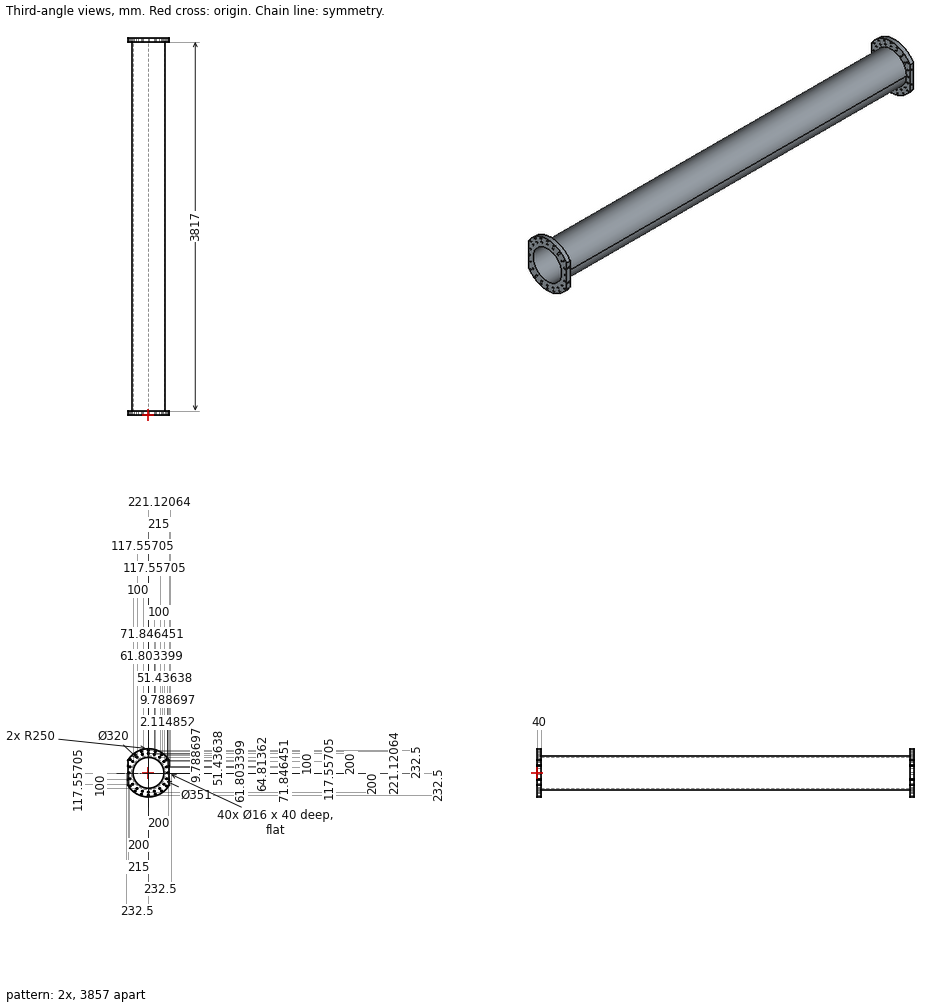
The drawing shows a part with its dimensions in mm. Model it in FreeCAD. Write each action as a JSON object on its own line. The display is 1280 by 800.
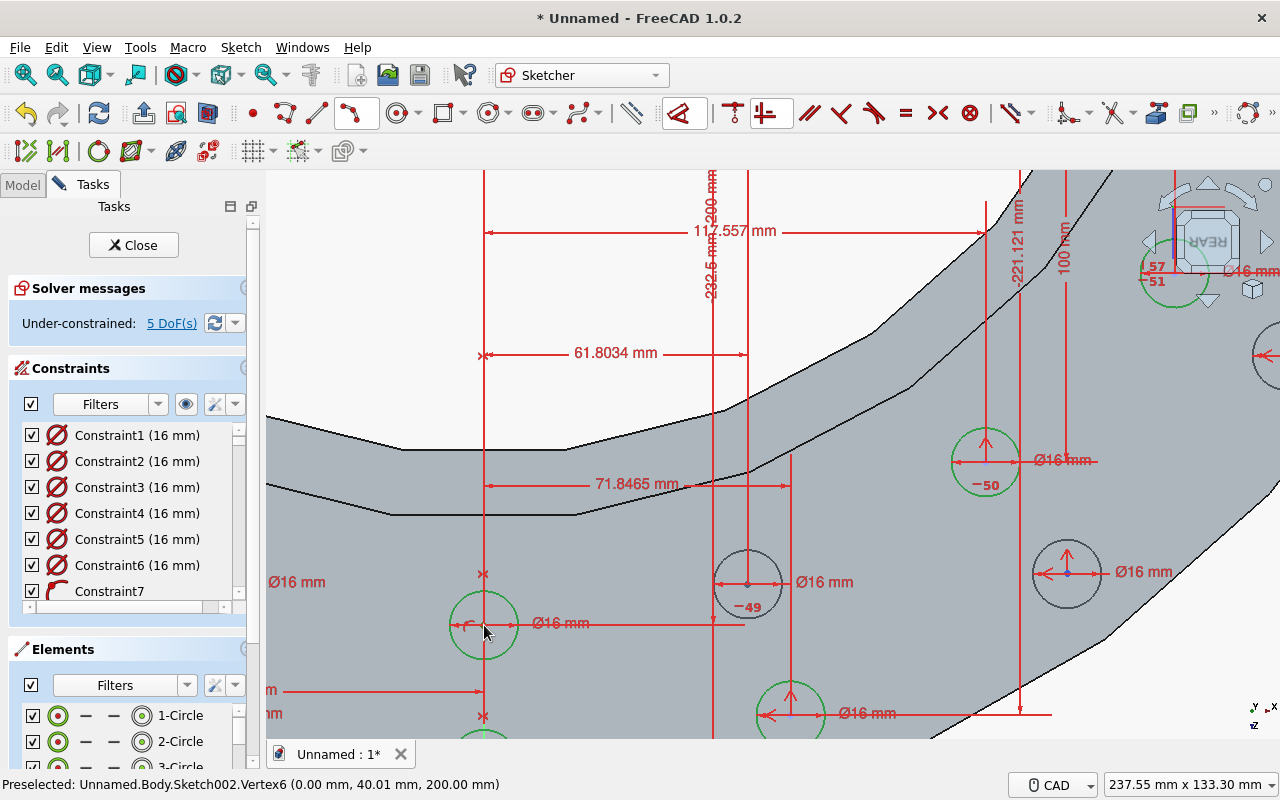
{"action": "key", "text": "i"}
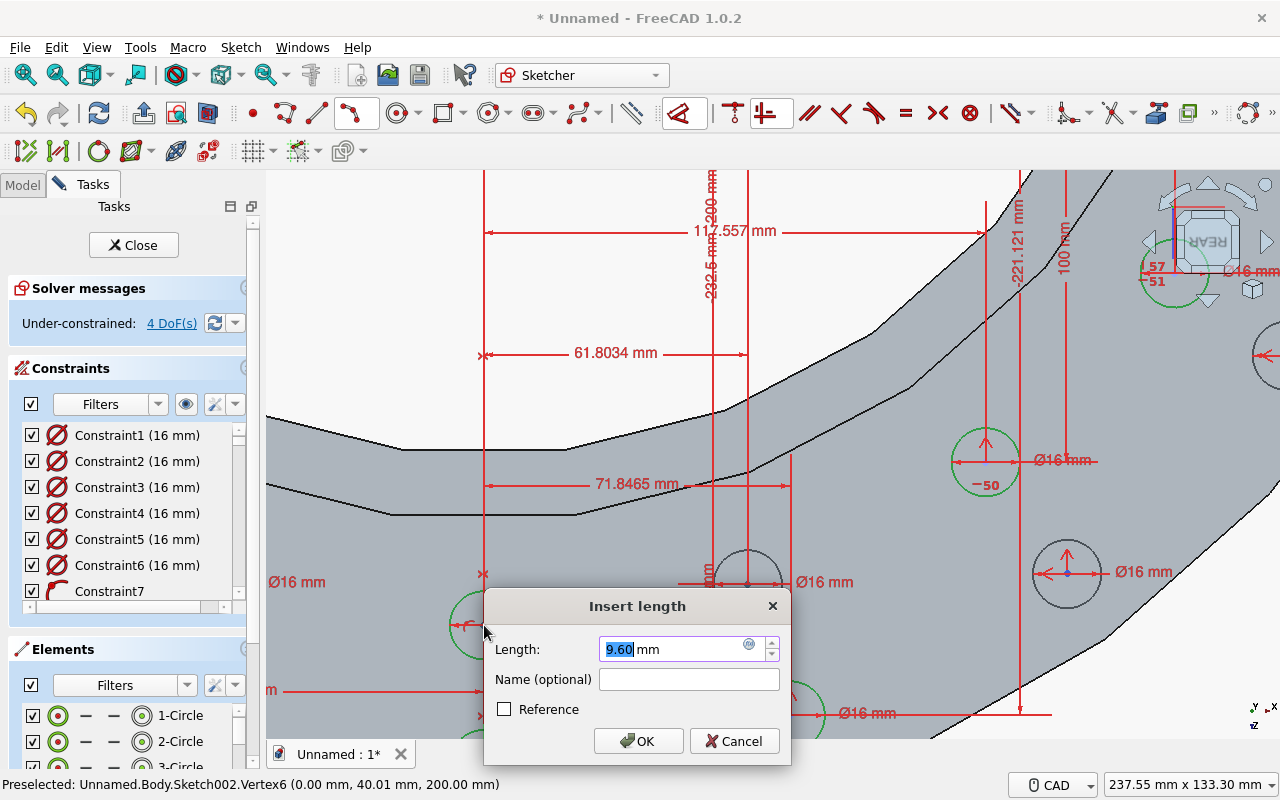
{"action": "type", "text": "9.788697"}
{"action": "key", "text": "Return"}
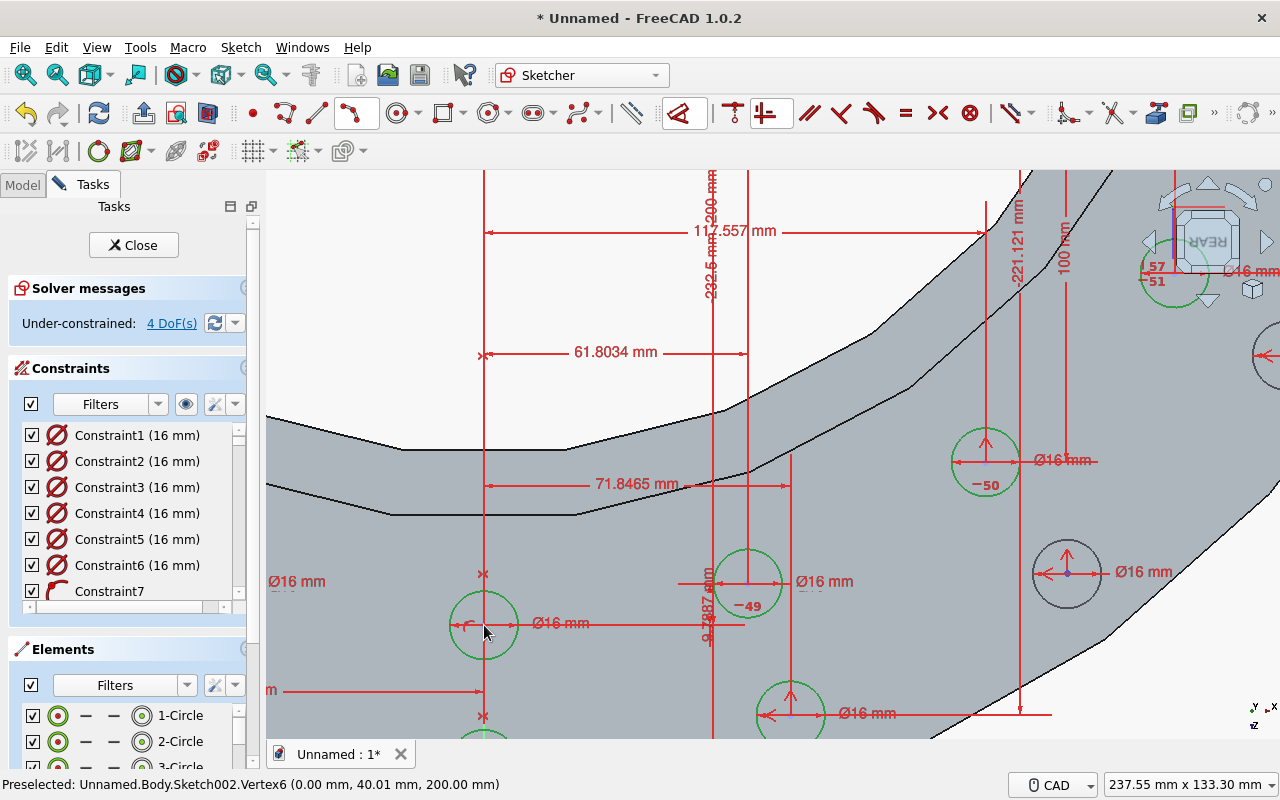
{"action": "scroll", "coordinate": [748, 590], "scroll_direction": "down", "scroll_amount": 9}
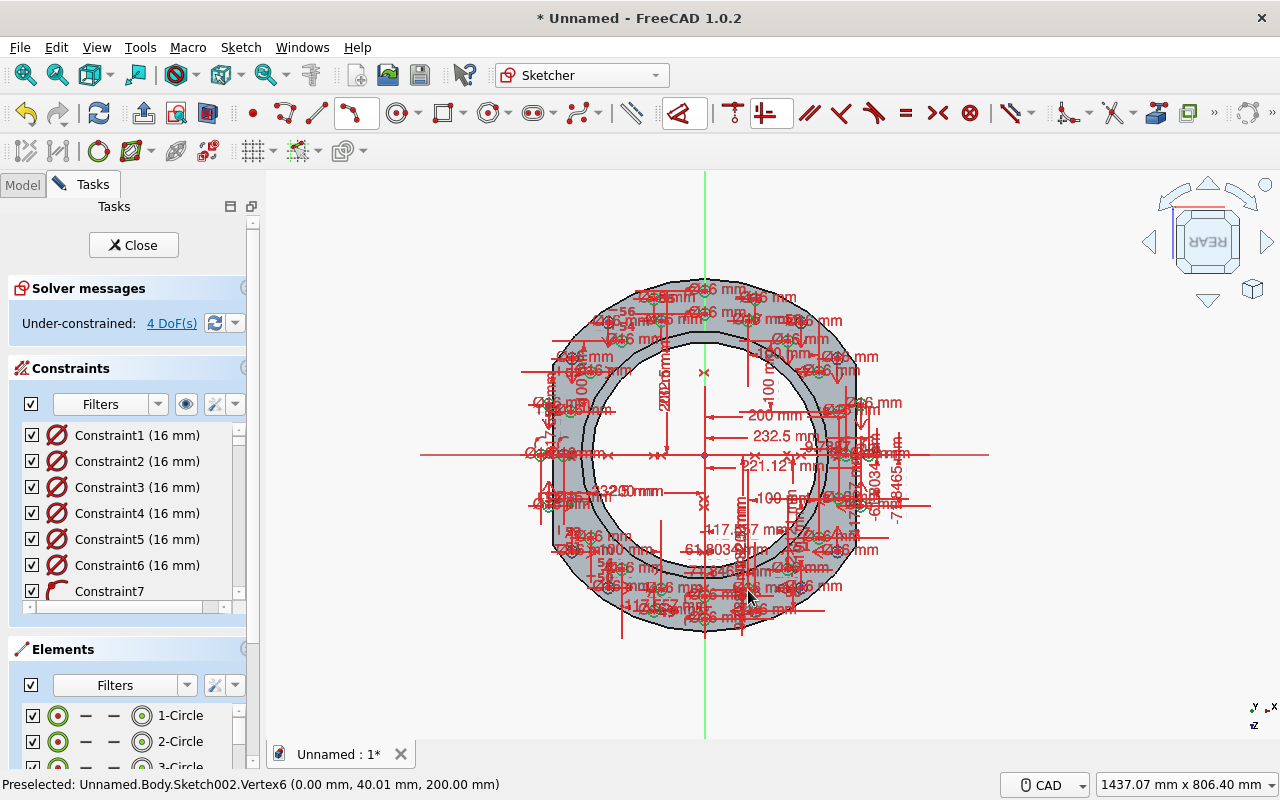
{"action": "scroll", "coordinate": [839, 499], "scroll_direction": "up", "scroll_amount": 17}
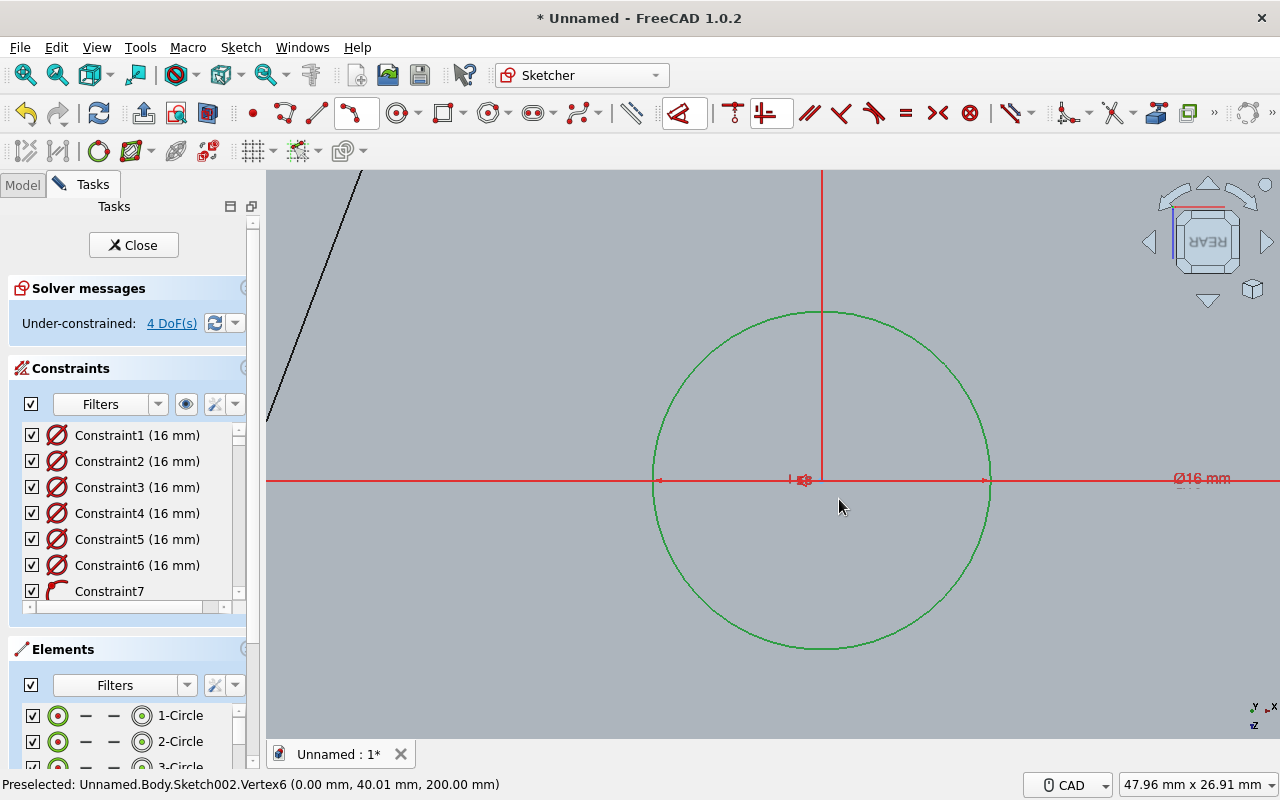
{"action": "left_click", "coordinate": [822, 481]}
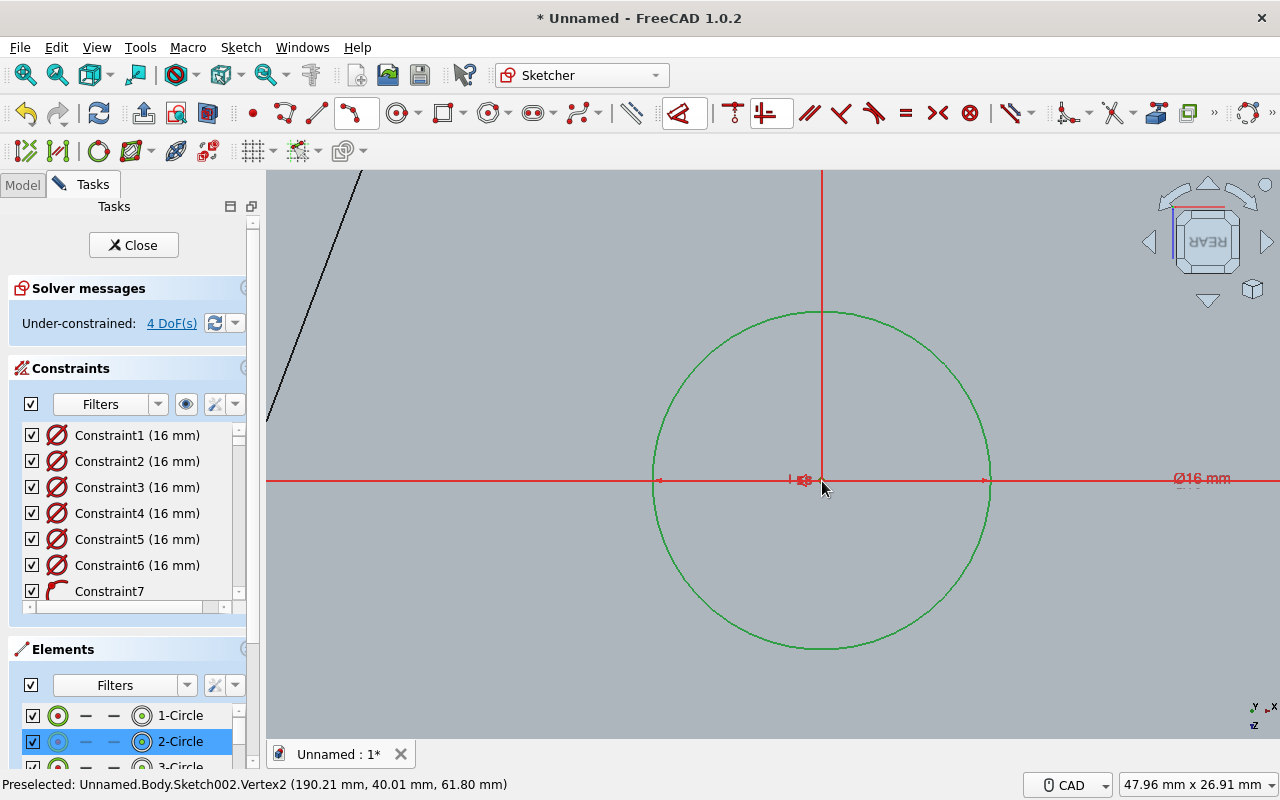
{"action": "scroll", "coordinate": [870, 509], "scroll_direction": "down", "scroll_amount": 16}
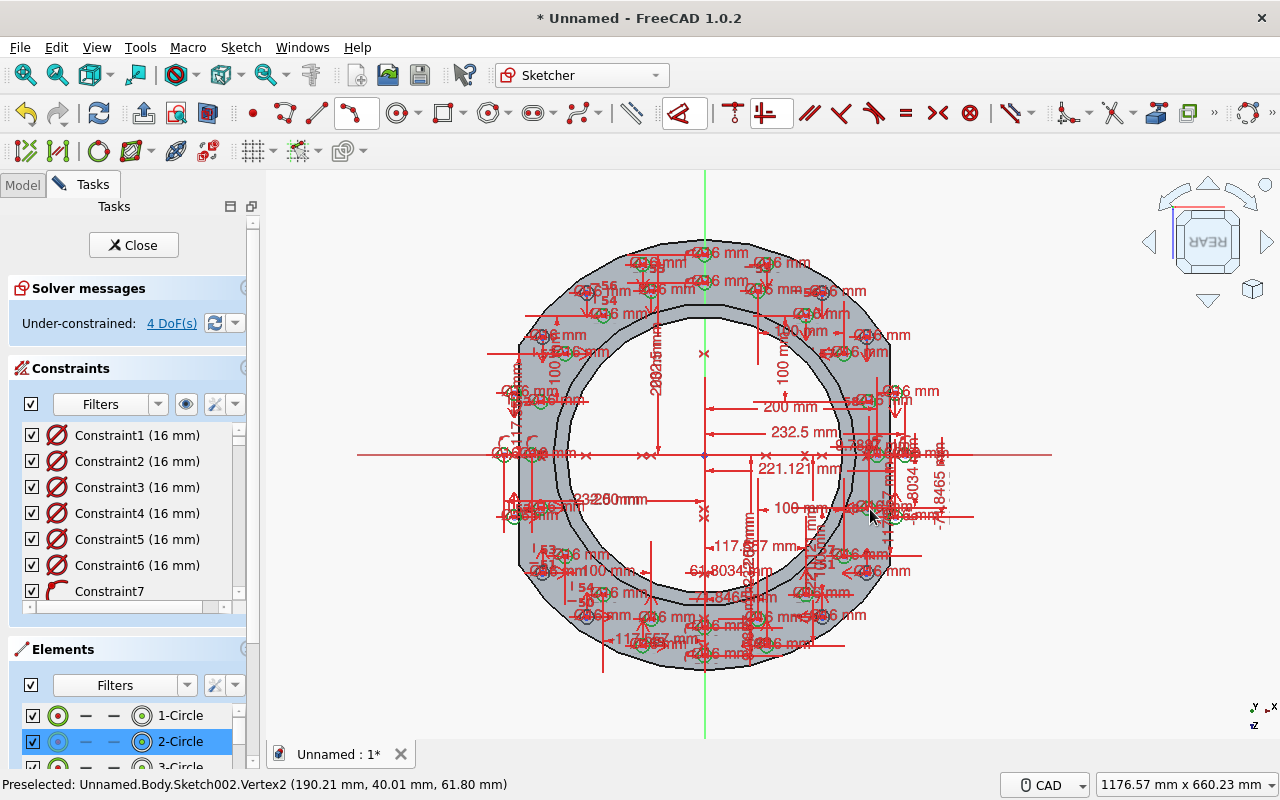
{"action": "scroll", "coordinate": [867, 573], "scroll_direction": "up", "scroll_amount": 16}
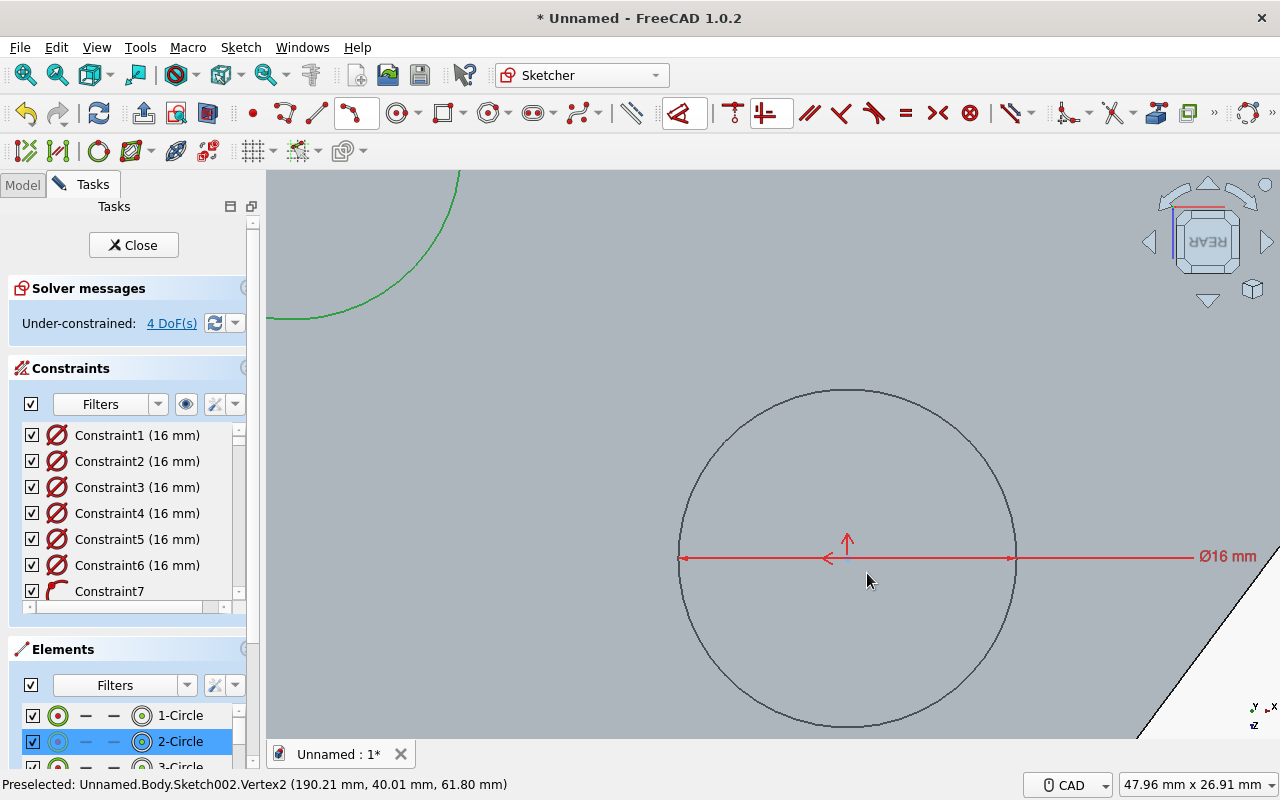
{"action": "left_click", "coordinate": [847, 558]}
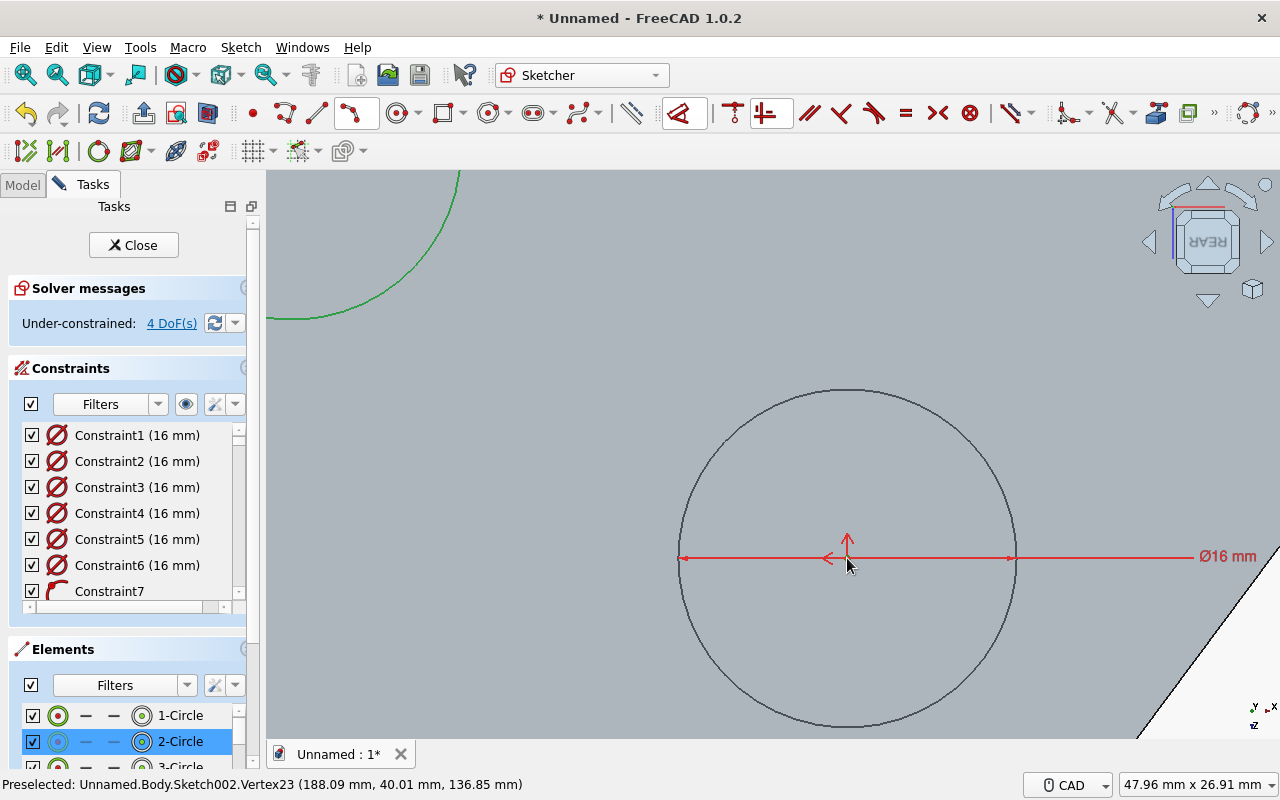
{"action": "key", "text": "l"}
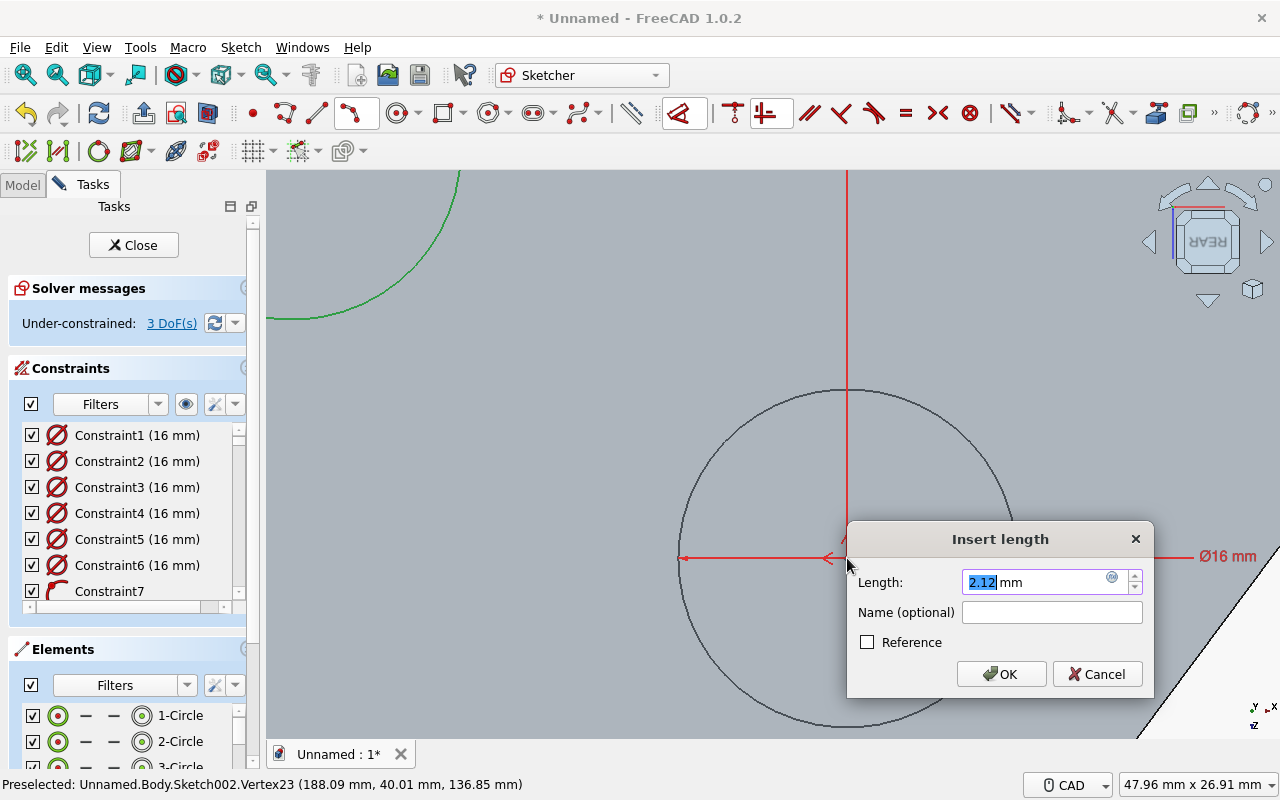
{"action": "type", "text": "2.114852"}
{"action": "key", "text": "Return"}